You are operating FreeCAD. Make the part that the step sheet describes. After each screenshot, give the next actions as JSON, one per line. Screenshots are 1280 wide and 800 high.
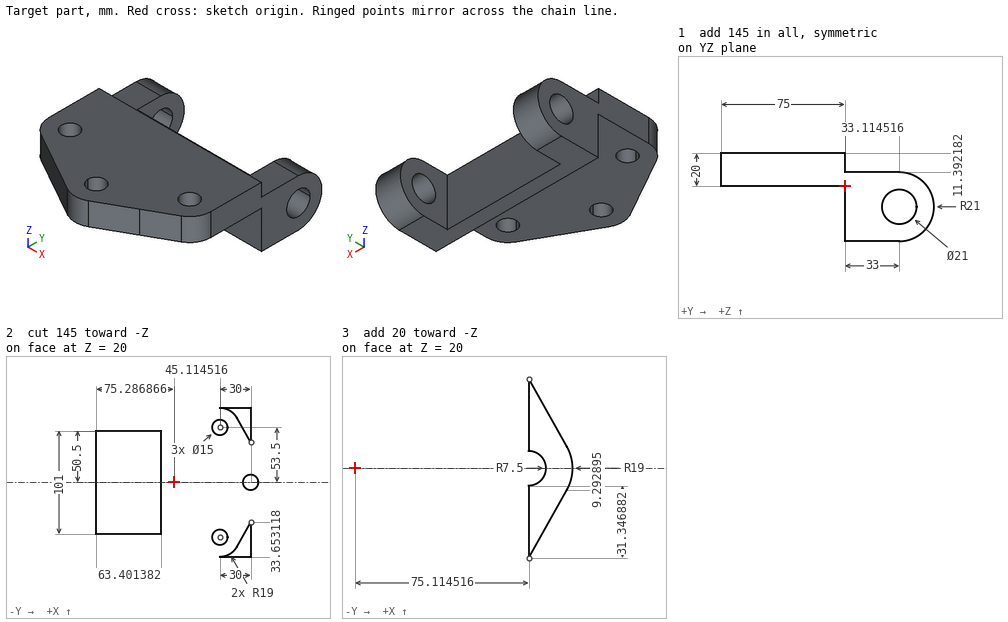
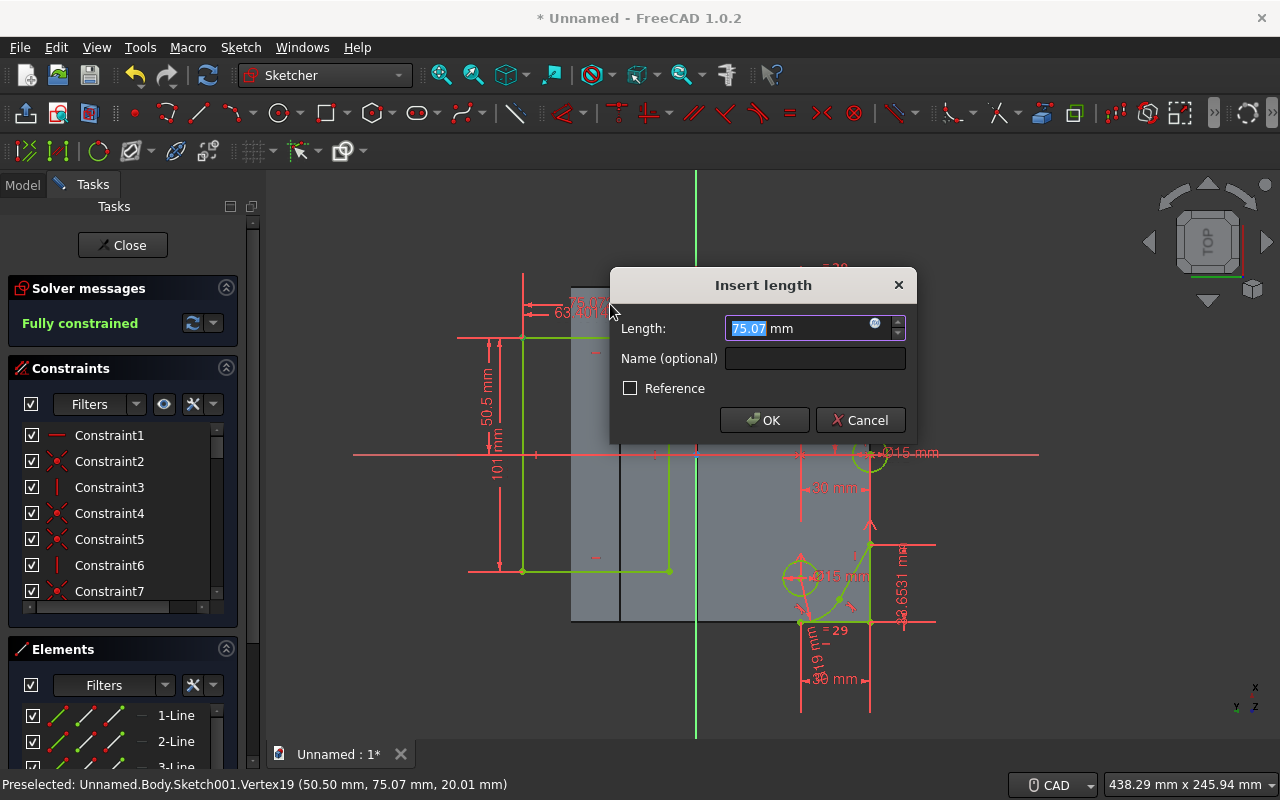
{"action": "type", "text": "75.286866"}
{"action": "key", "text": "Return"}
{"action": "key", "text": "Escape"}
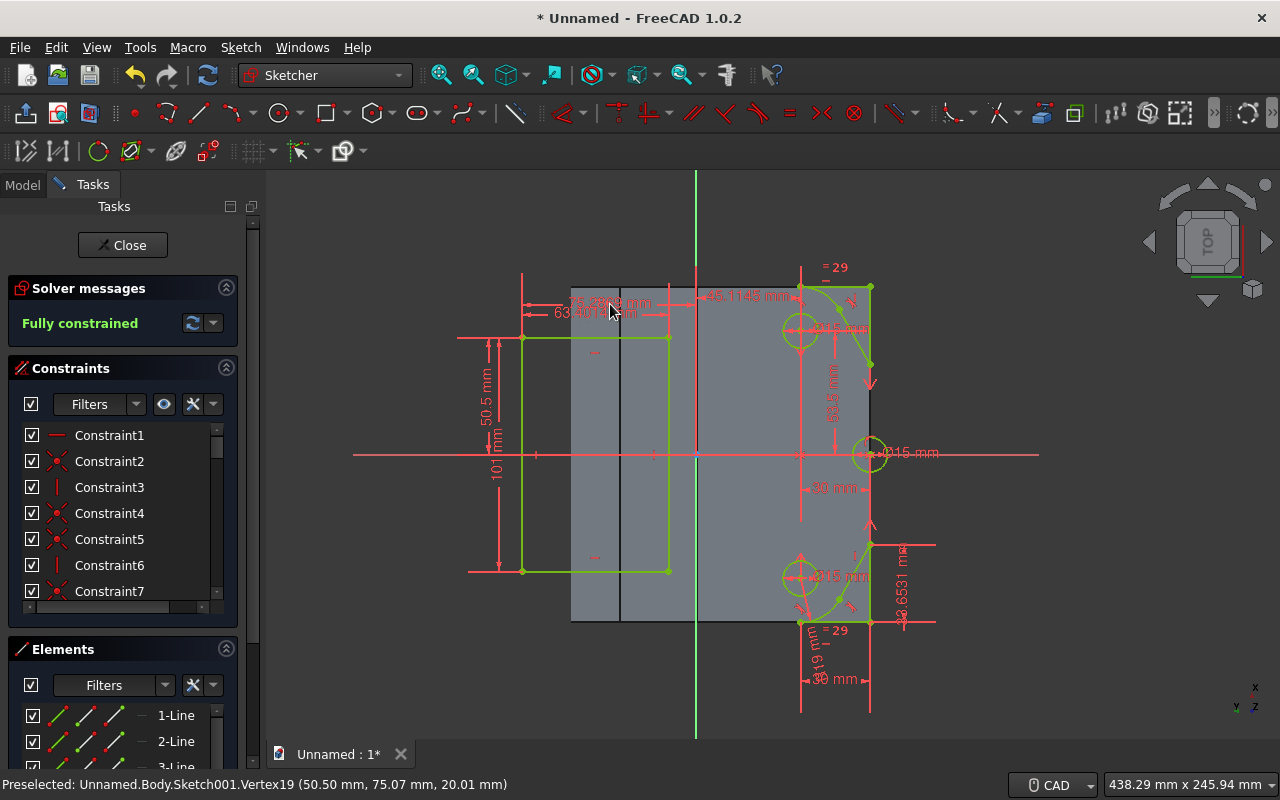
{"action": "left_click", "coordinate": [123, 245]}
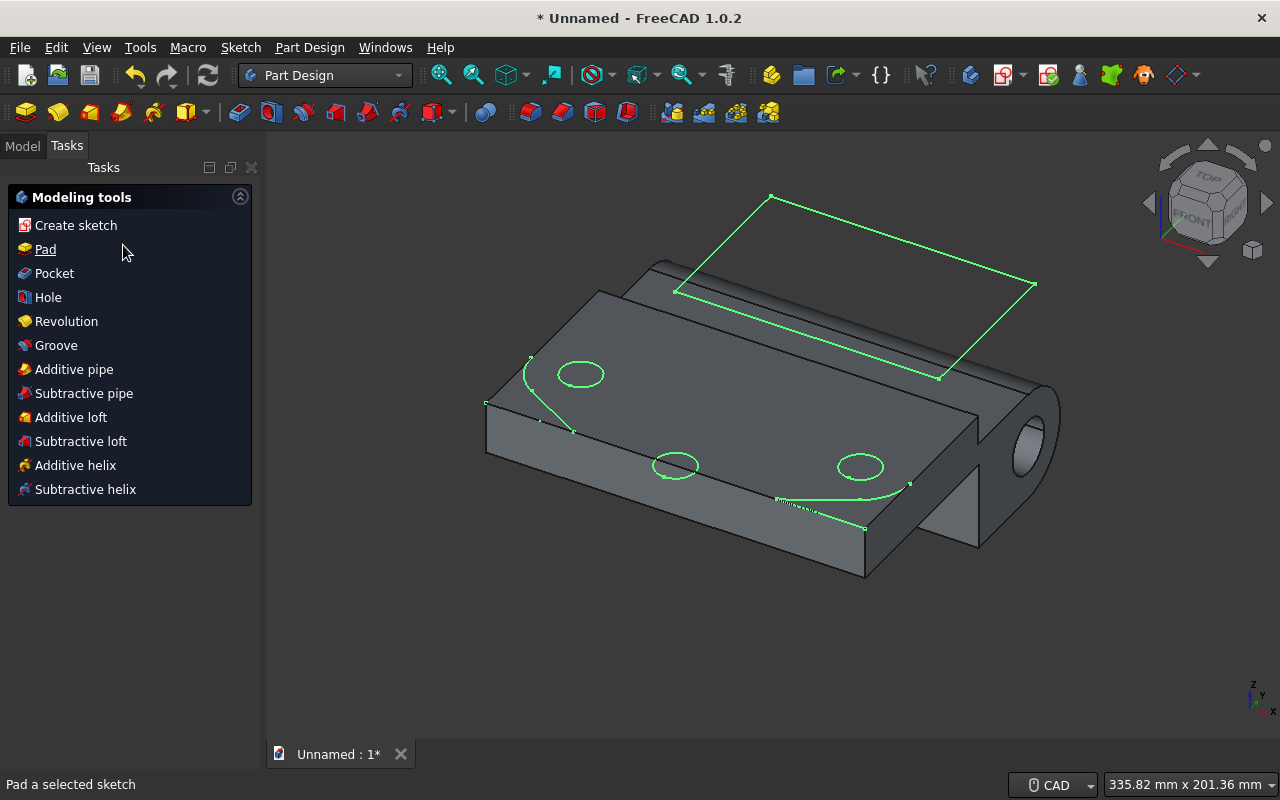
{"action": "left_click", "coordinate": [240, 112]}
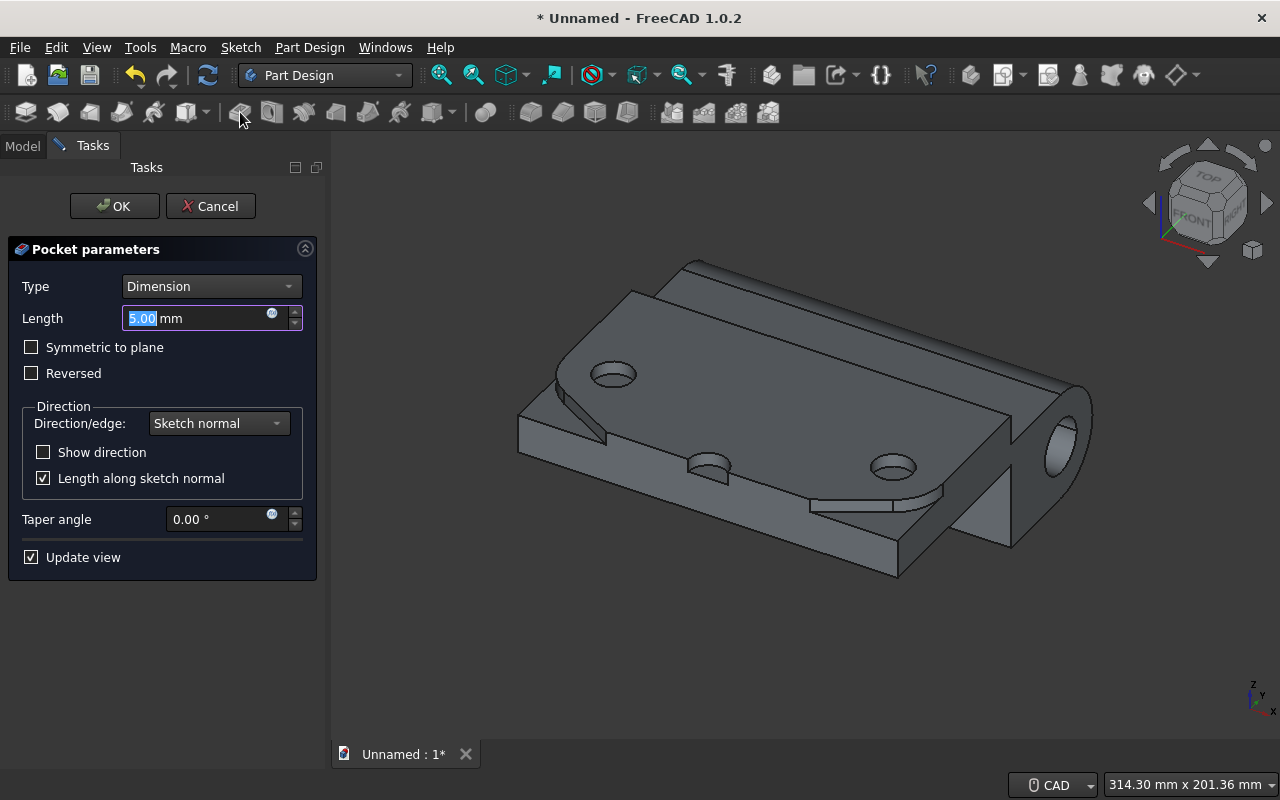
{"action": "type", "text": "145"}
{"action": "key", "text": "Tab"}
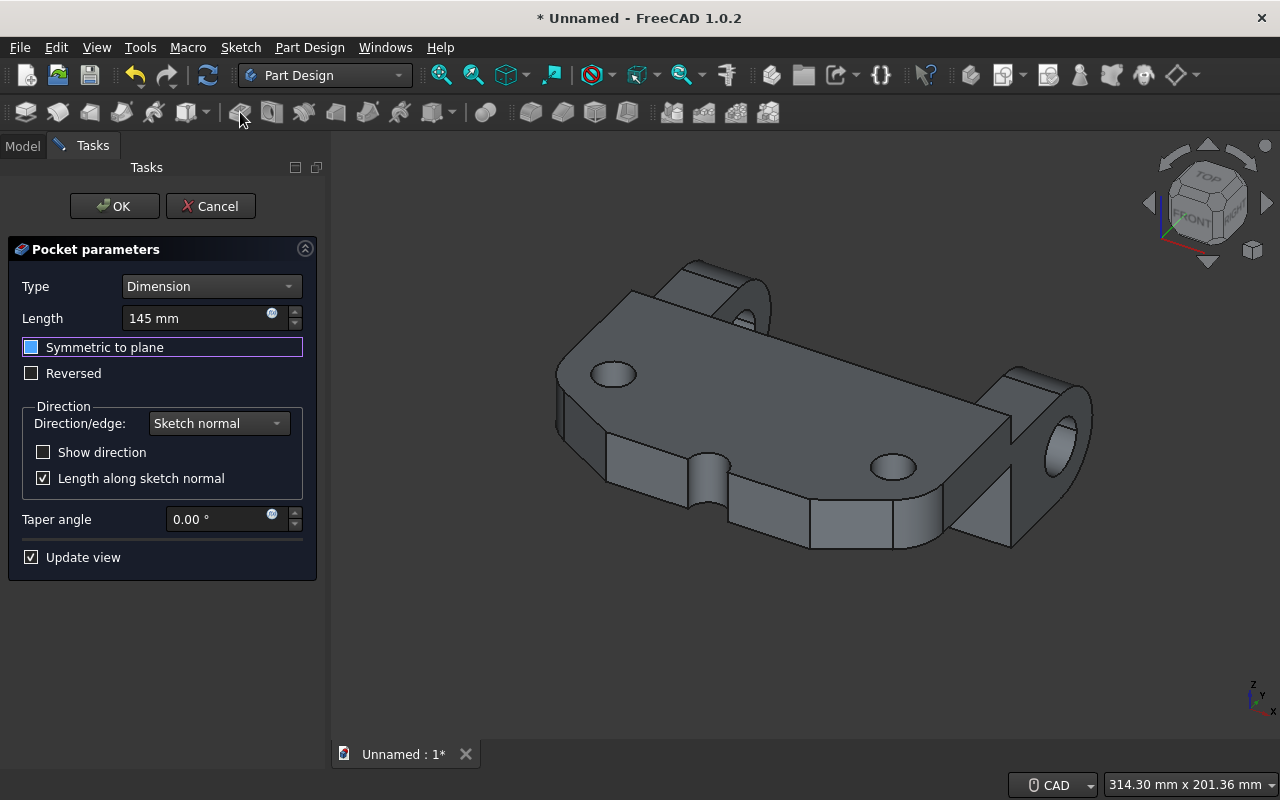
{"action": "left_click", "coordinate": [115, 206]}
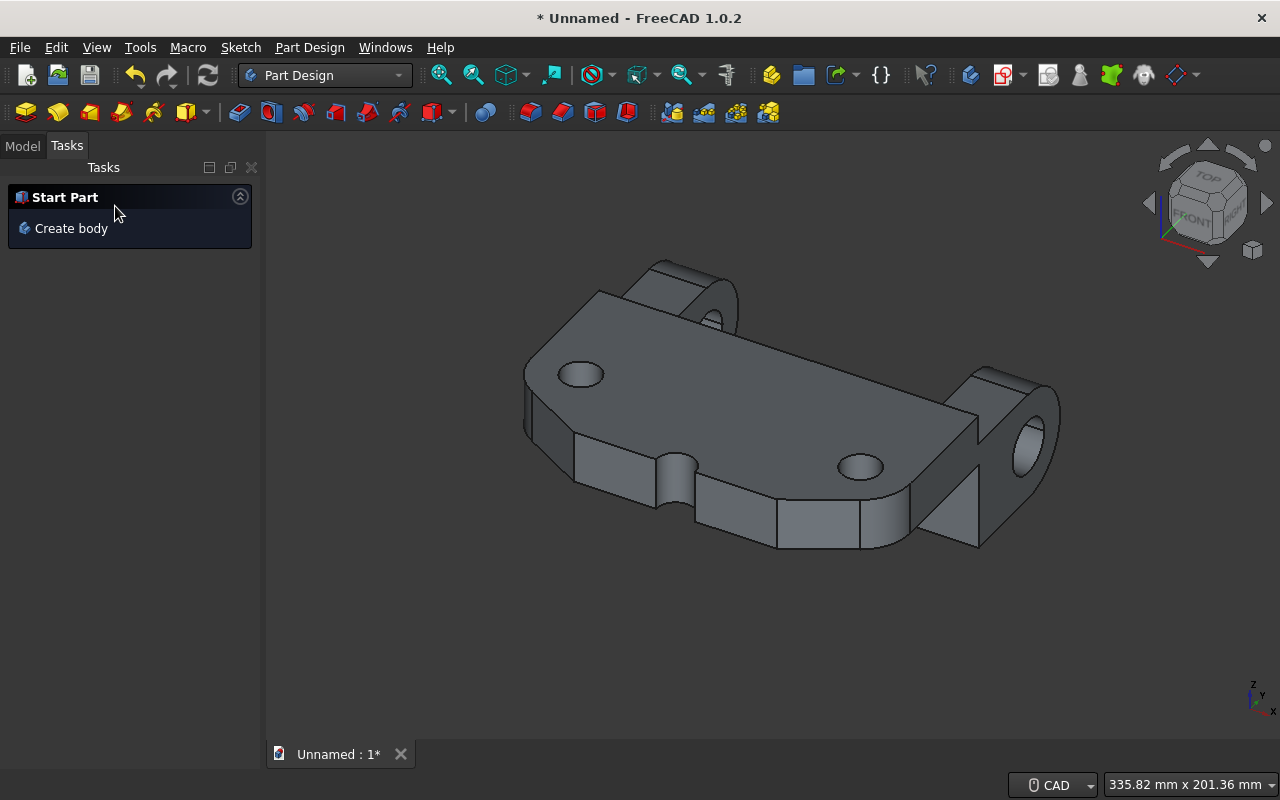
{"action": "left_click", "coordinate": [732, 409]}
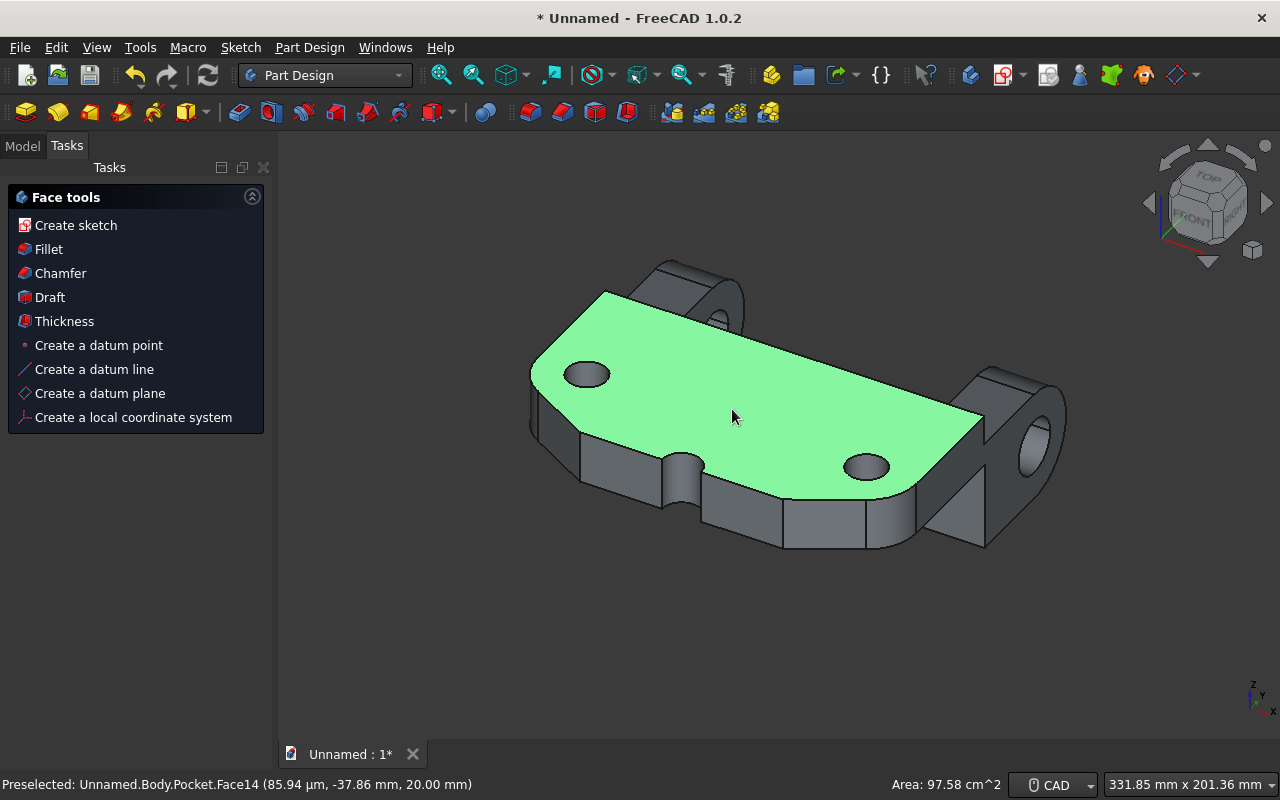
{"action": "left_click", "coordinate": [1004, 76]}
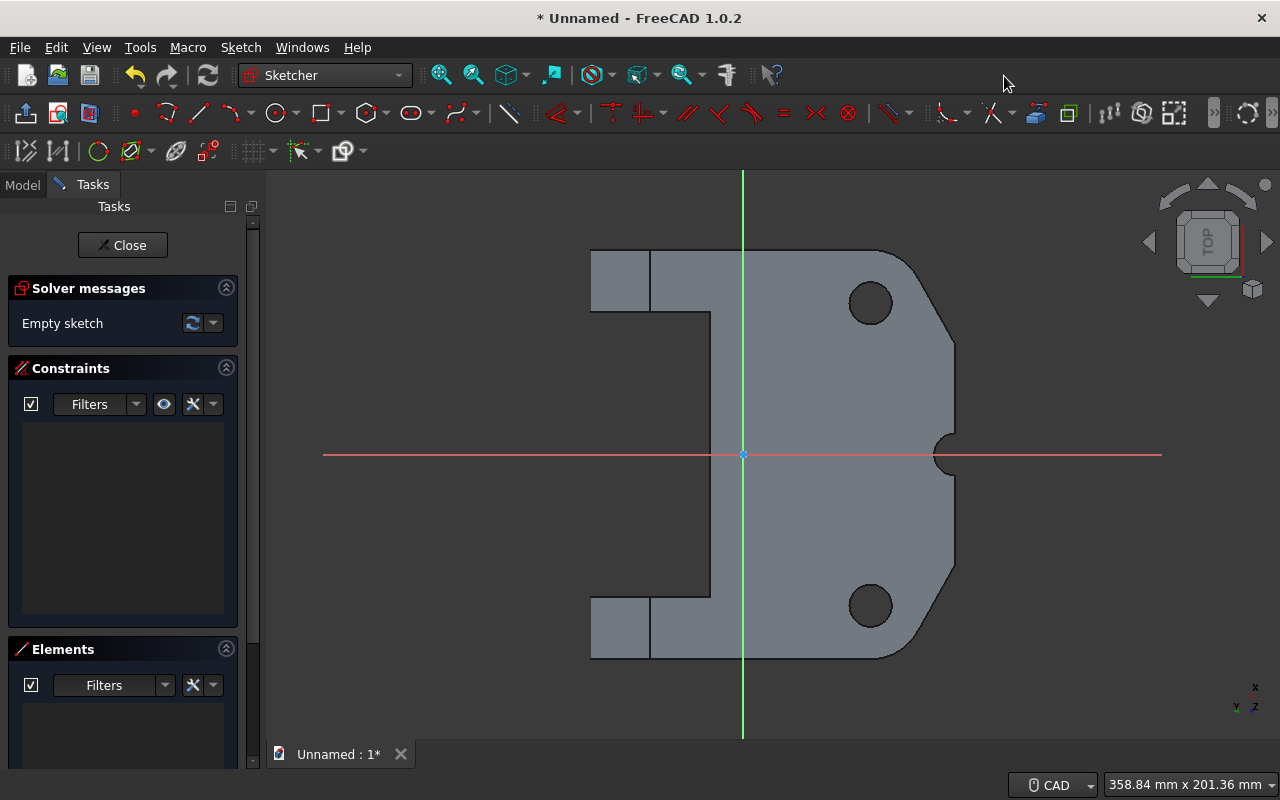
{"action": "scroll", "coordinate": [1085, 454], "scroll_direction": "up", "scroll_amount": 3}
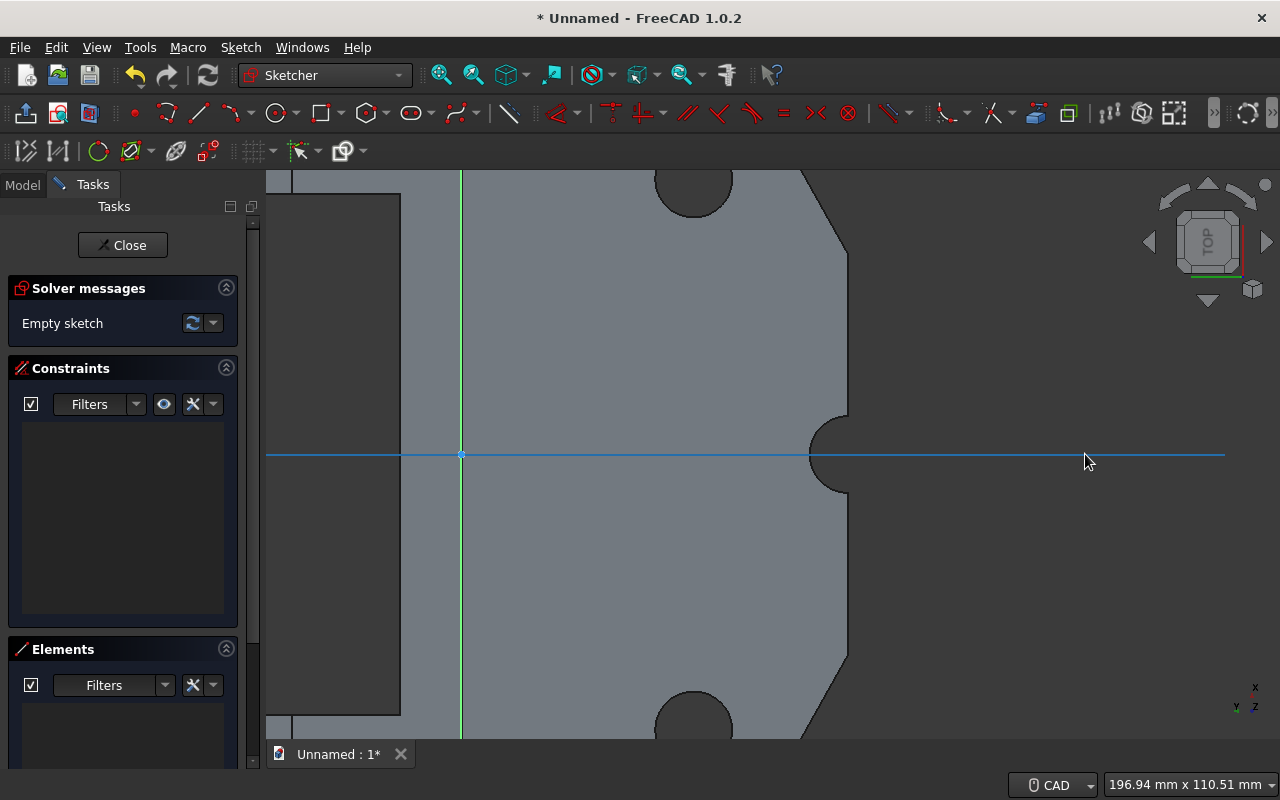
{"action": "left_click", "coordinate": [168, 114]}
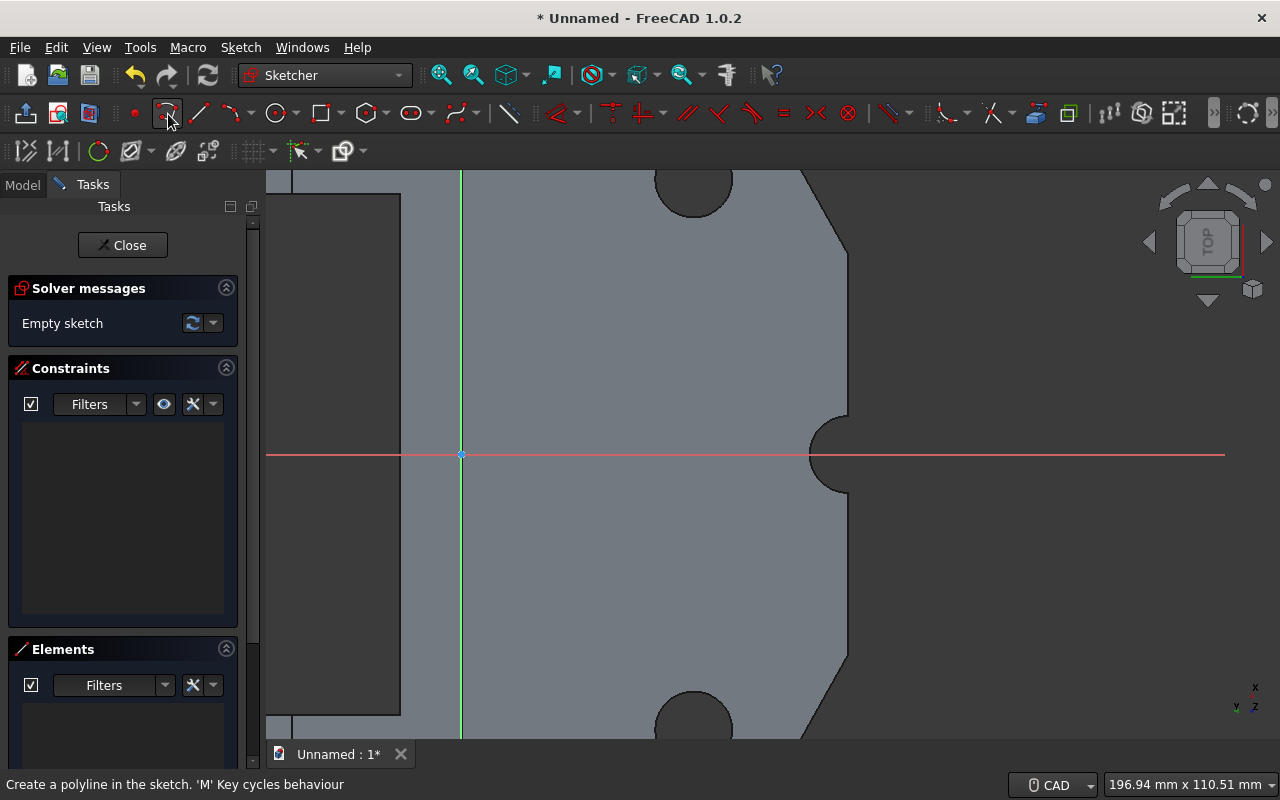
{"action": "left_click", "coordinate": [848, 493]}
{"action": "left_click", "coordinate": [848, 655]}
{"action": "left_click", "coordinate": [934, 502]}
{"action": "right_click", "coordinate": [934, 502]}